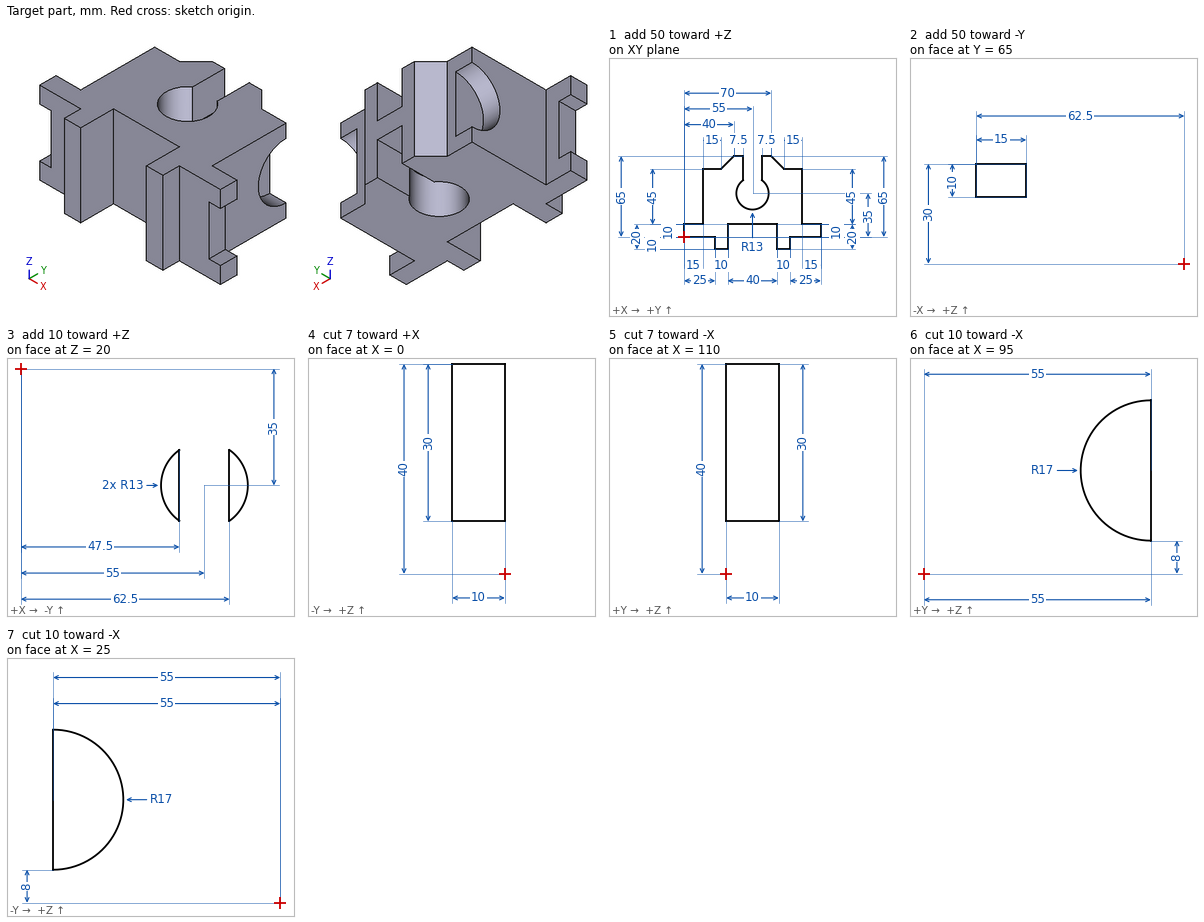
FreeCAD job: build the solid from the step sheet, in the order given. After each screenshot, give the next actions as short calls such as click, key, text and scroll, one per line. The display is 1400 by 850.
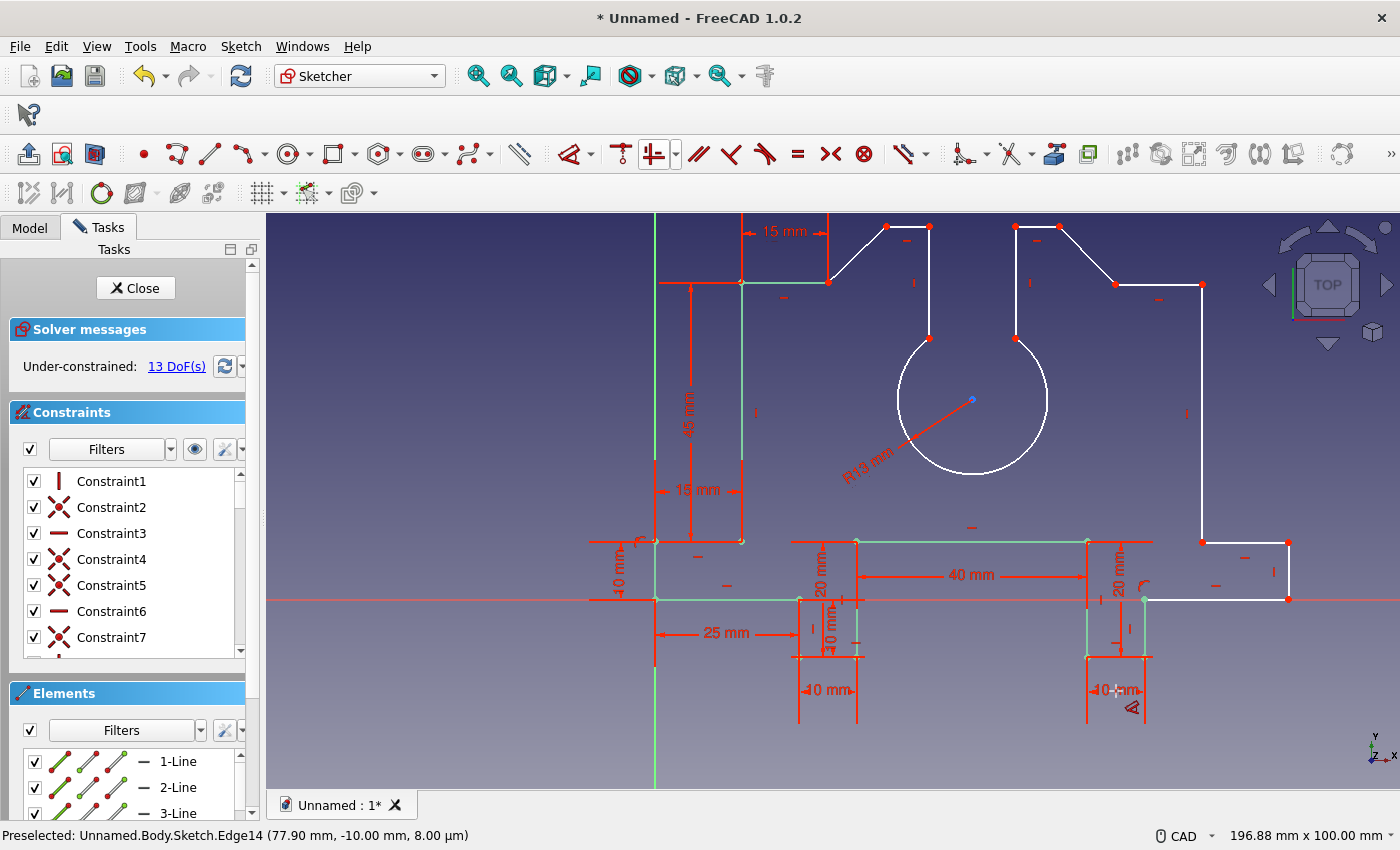
click(1188, 600)
click(1190, 634)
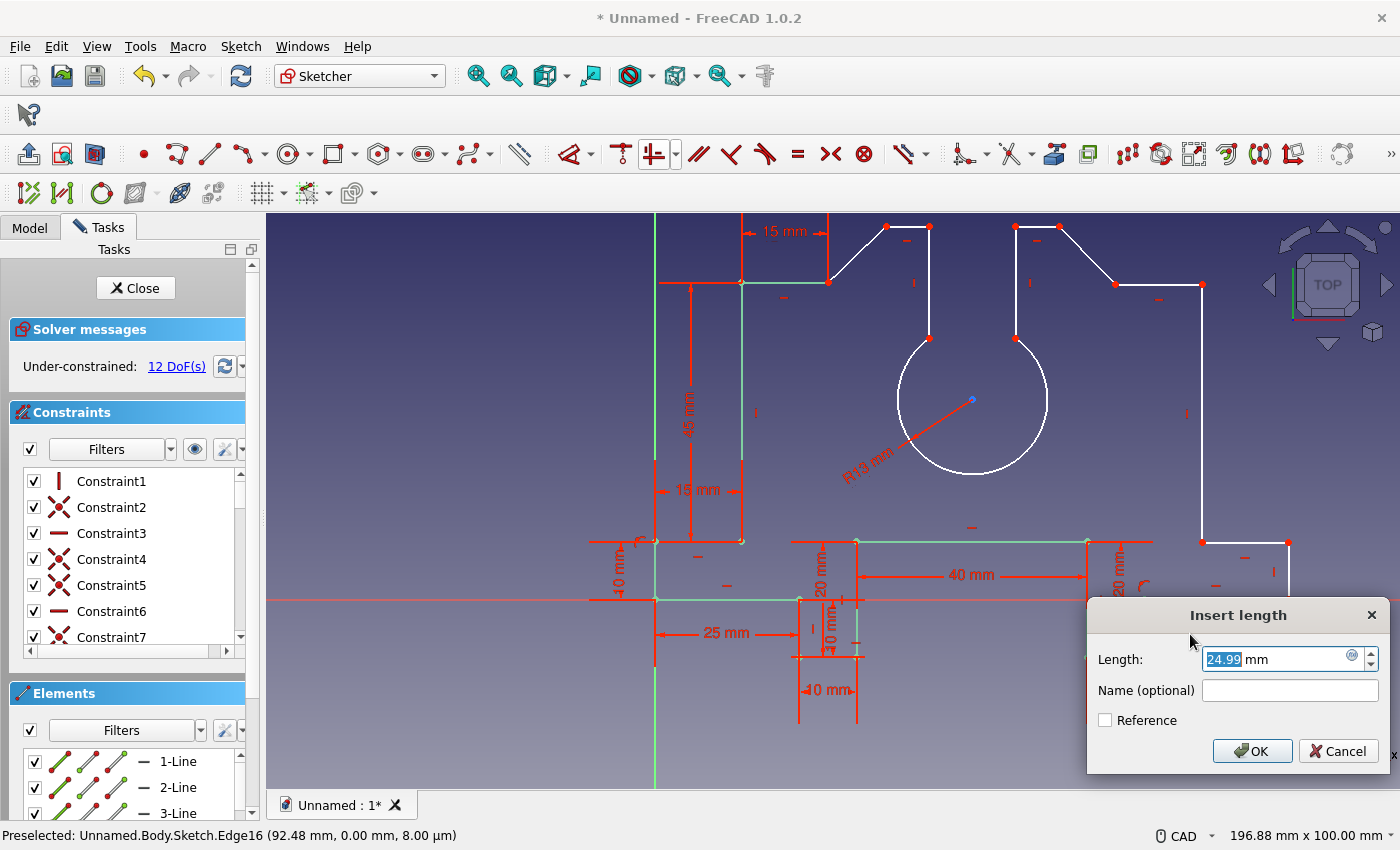
text(25)
key(Return)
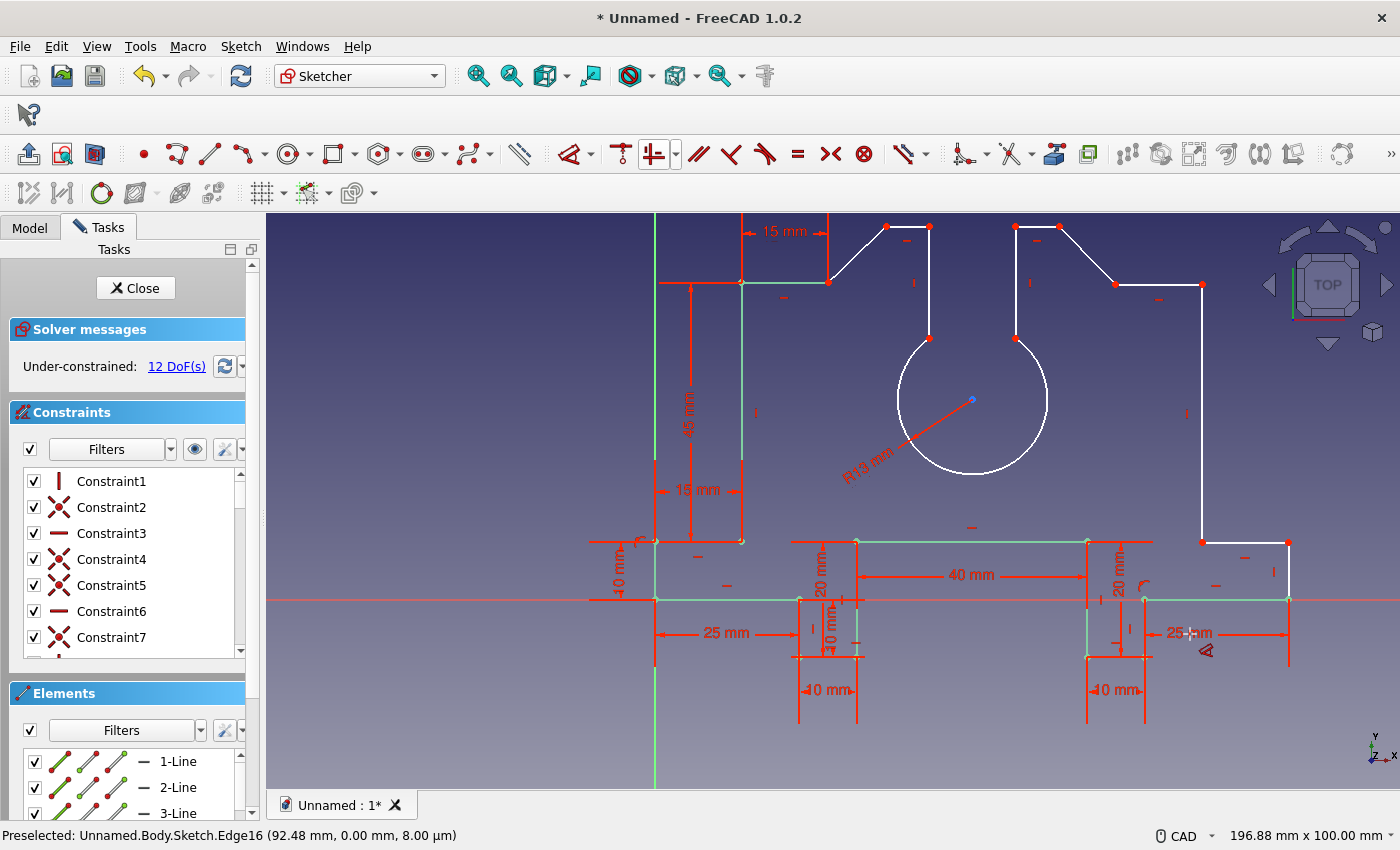
scroll(294, 761, down, 1)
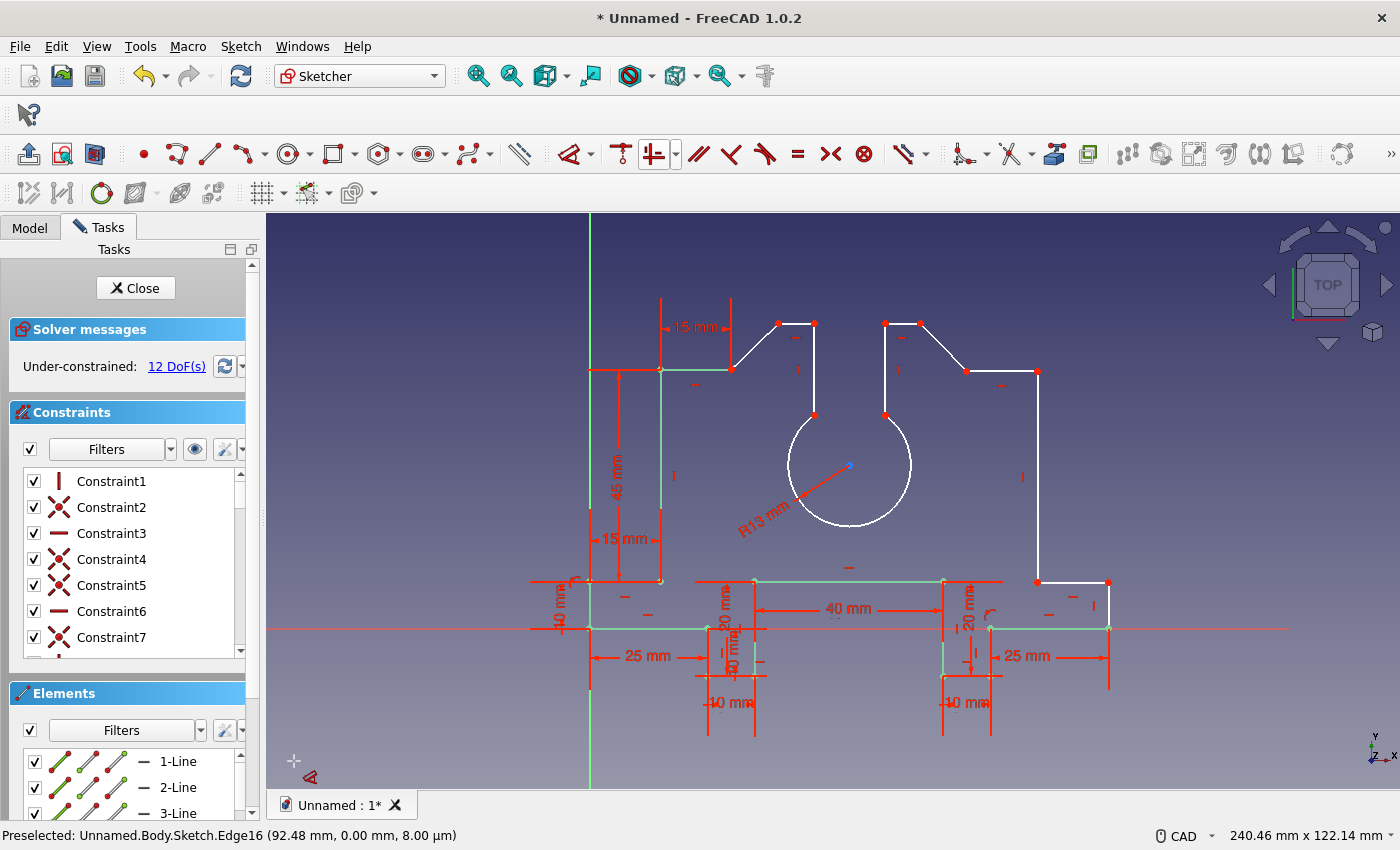
click(1109, 615)
click(1143, 606)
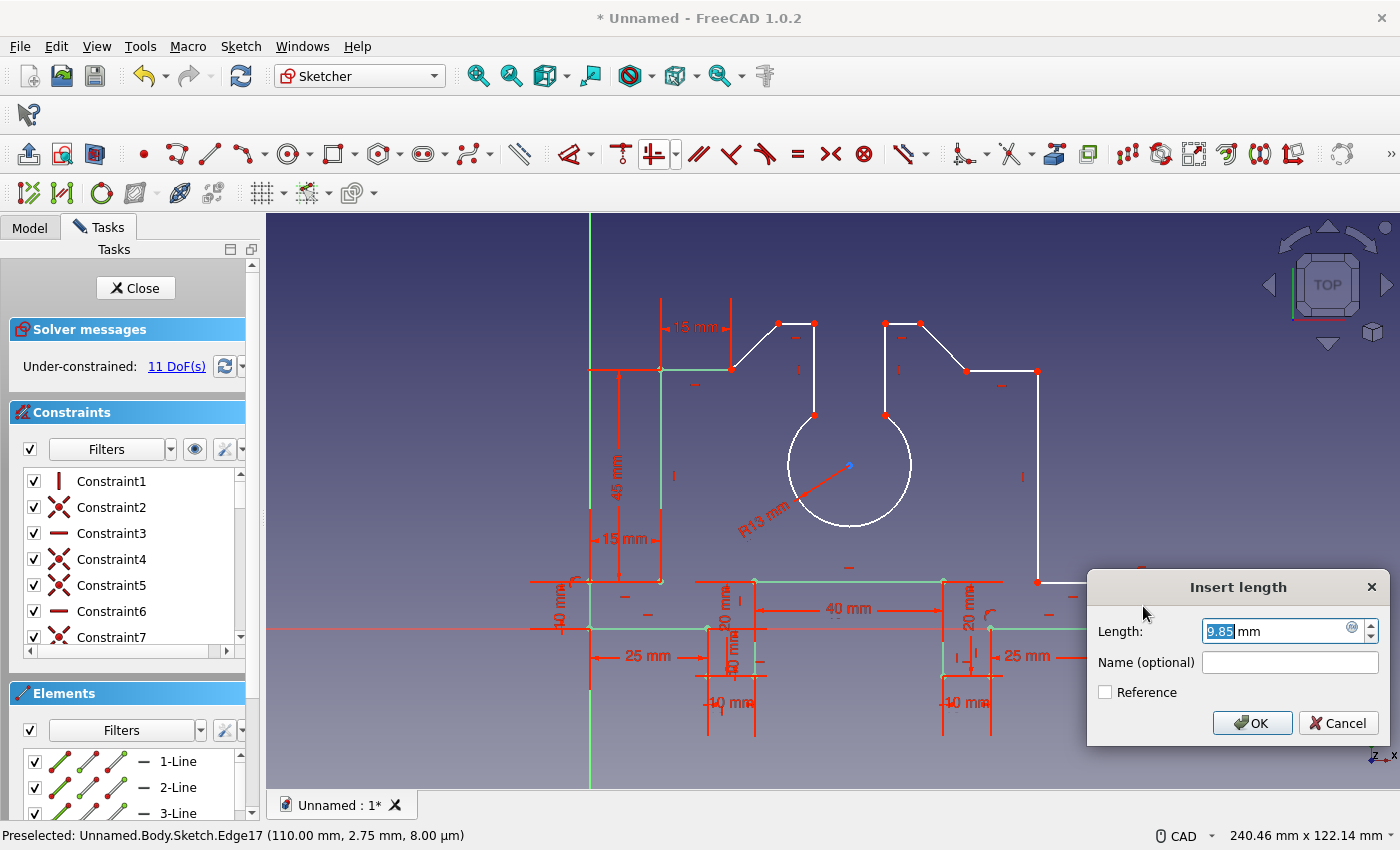
text(10)
key(Return)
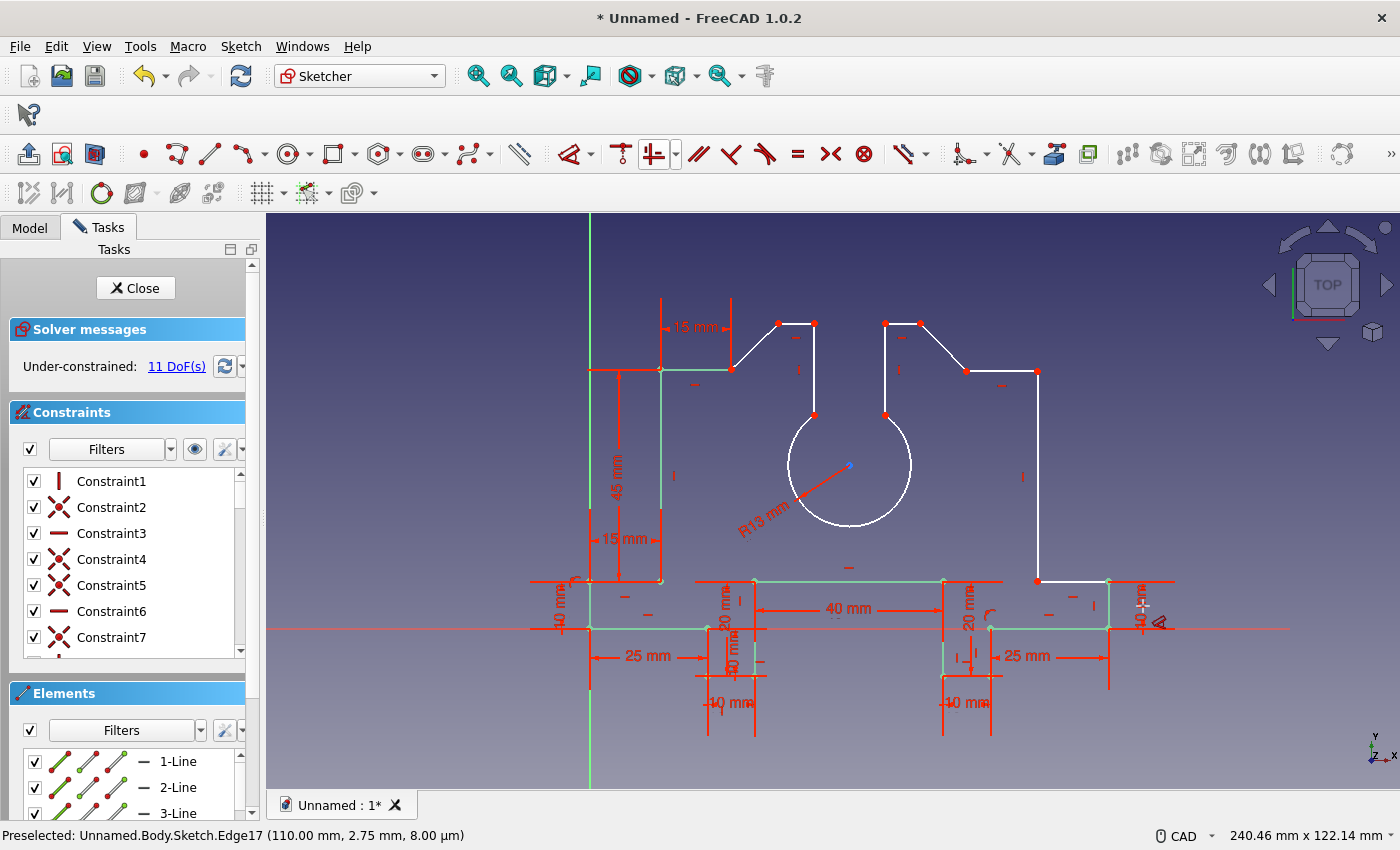
click(1087, 582)
click(1057, 616)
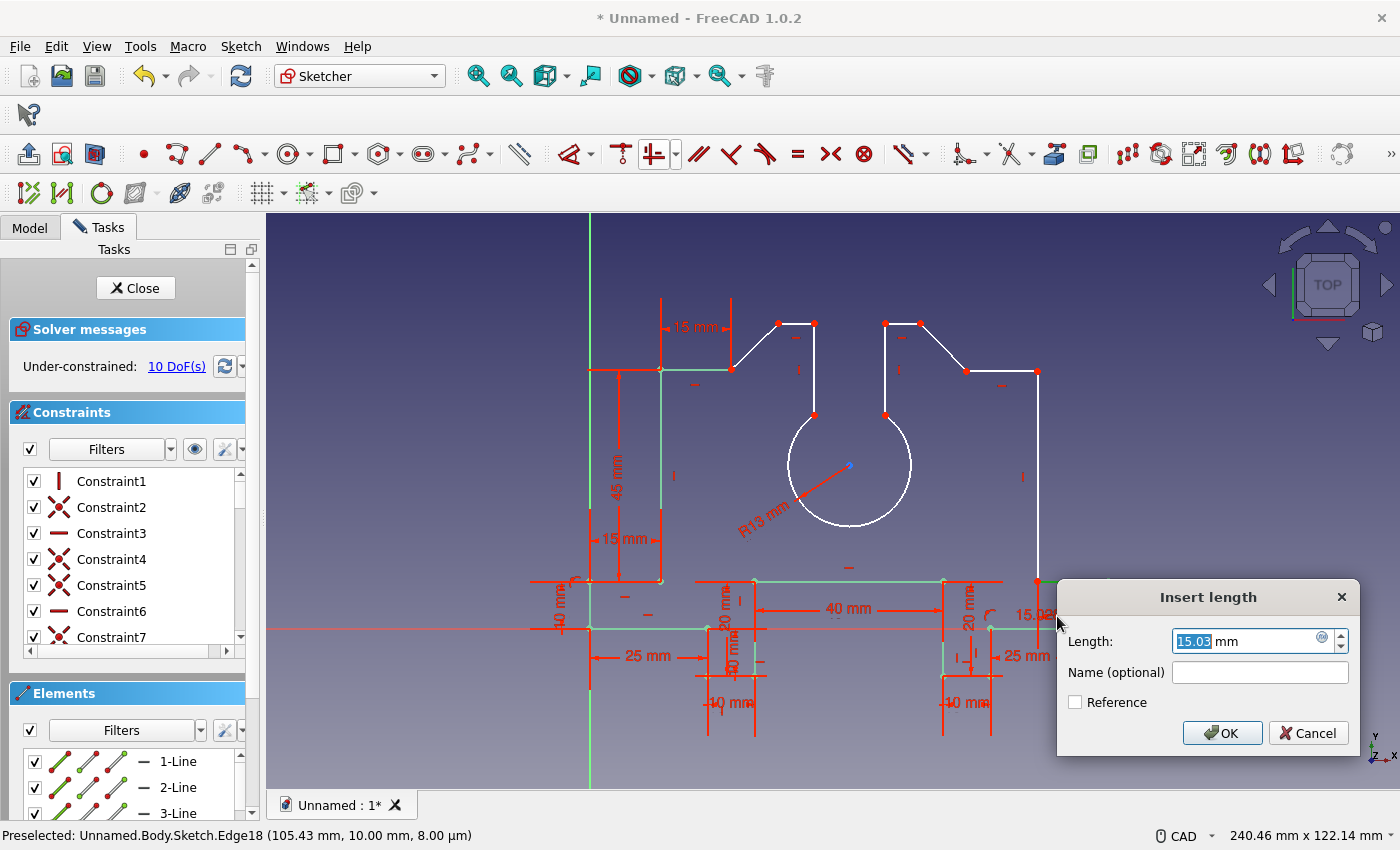
text(15)
key(Return)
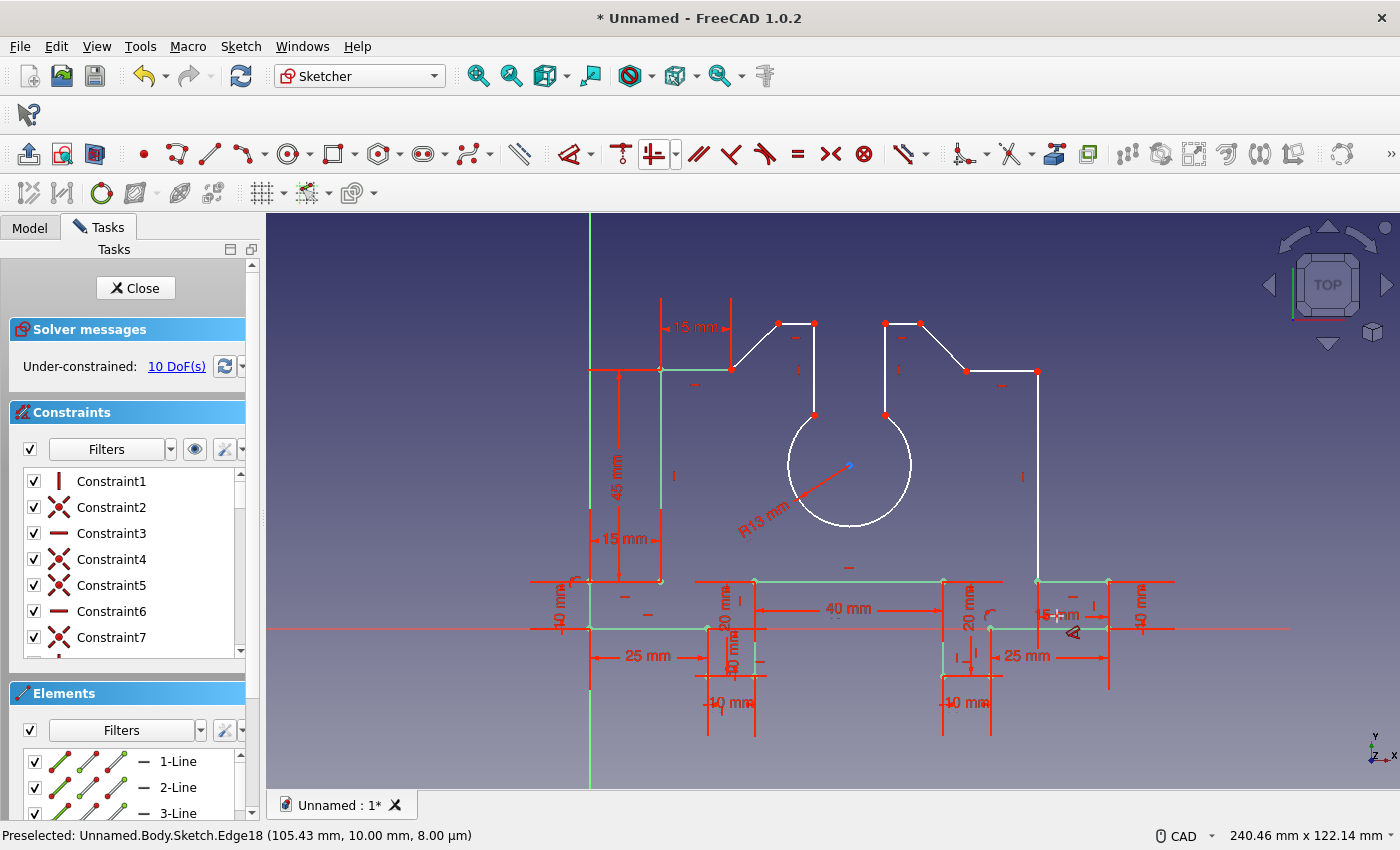
click(1038, 519)
click(1072, 477)